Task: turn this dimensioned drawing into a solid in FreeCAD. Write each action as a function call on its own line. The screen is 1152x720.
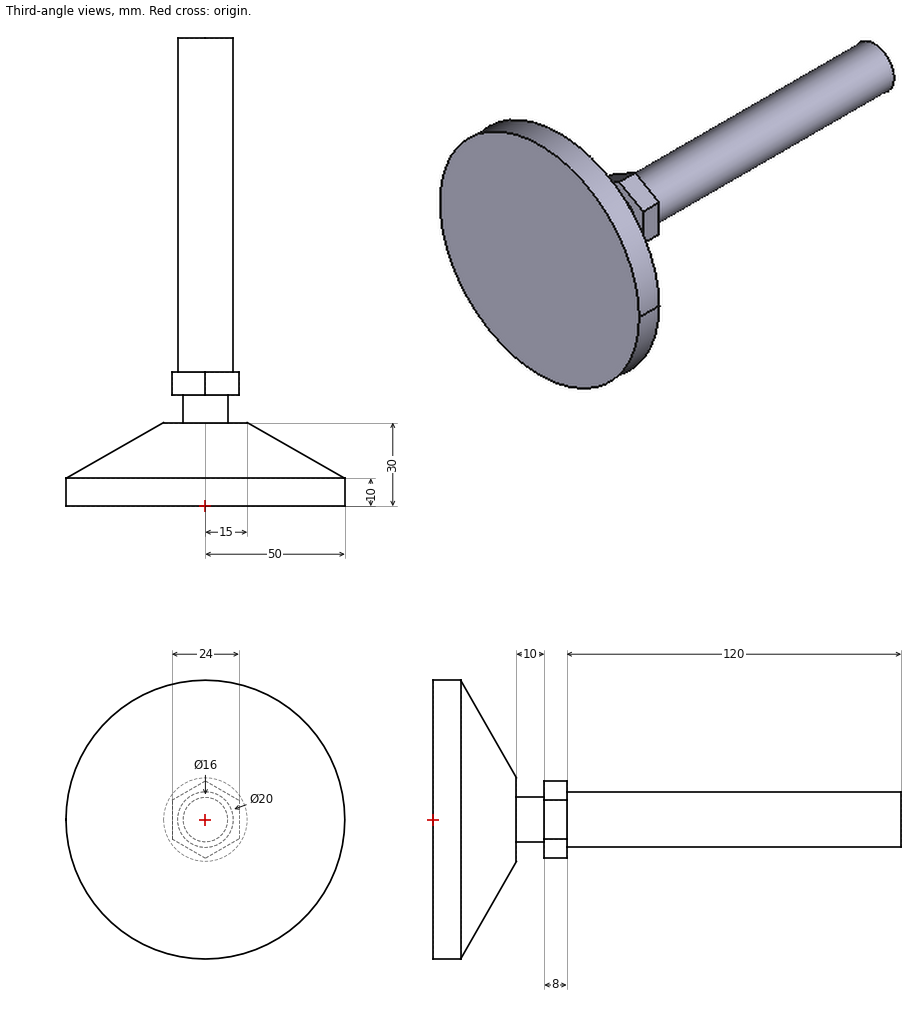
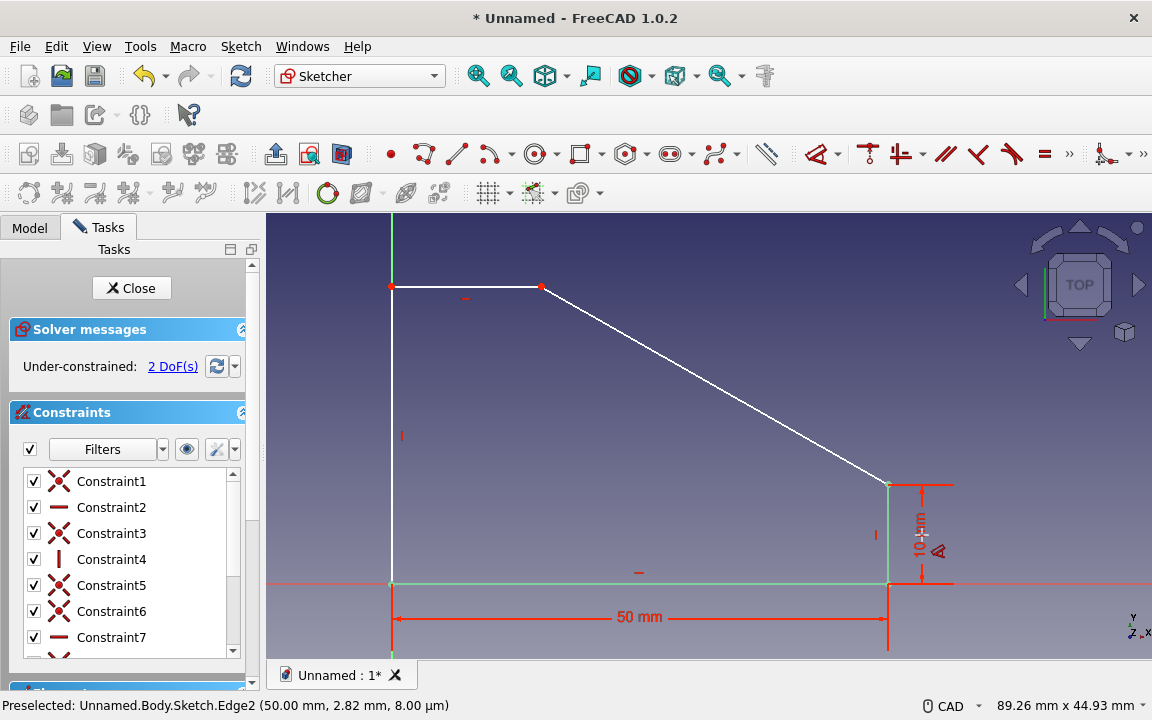
click(496, 287)
click(466, 253)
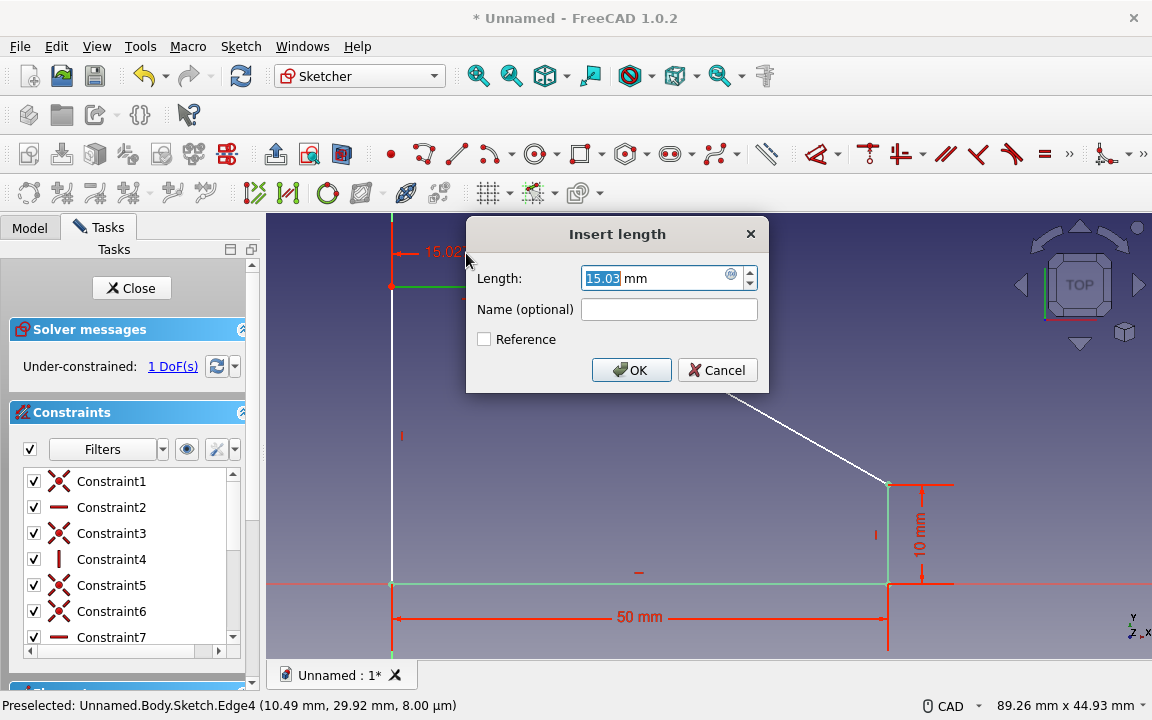
text(15)
key(Return)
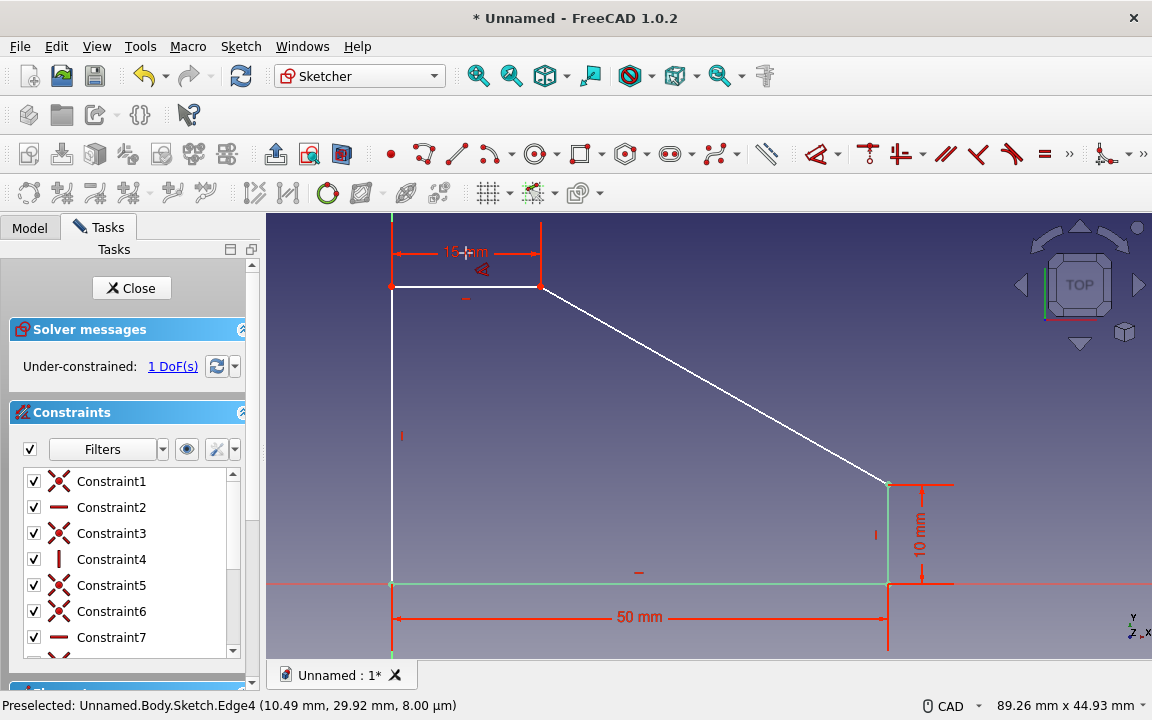
click(392, 376)
click(358, 436)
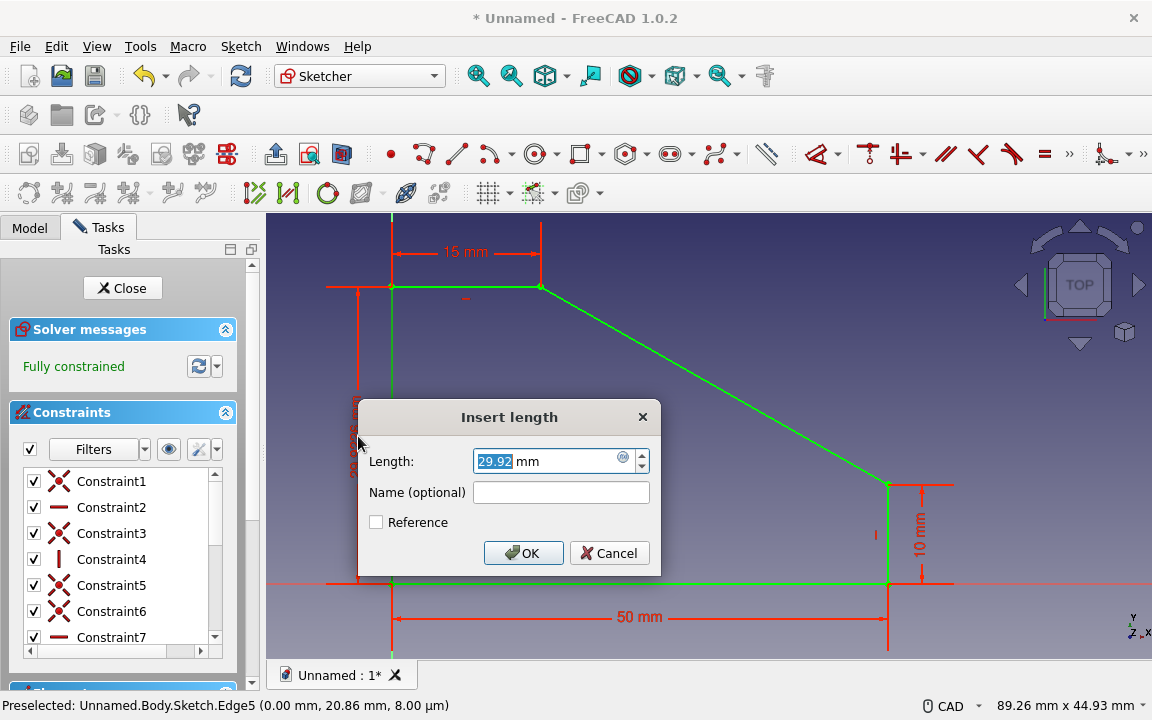
text(30)
key(Return)
key(Escape)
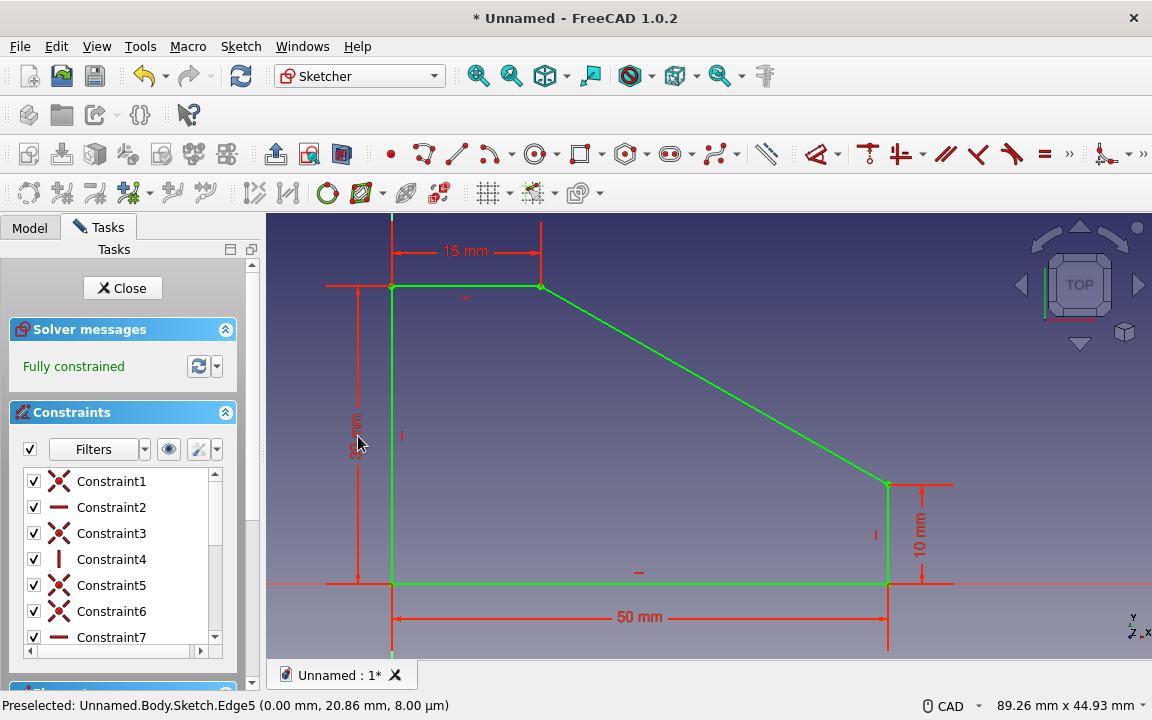
click(123, 288)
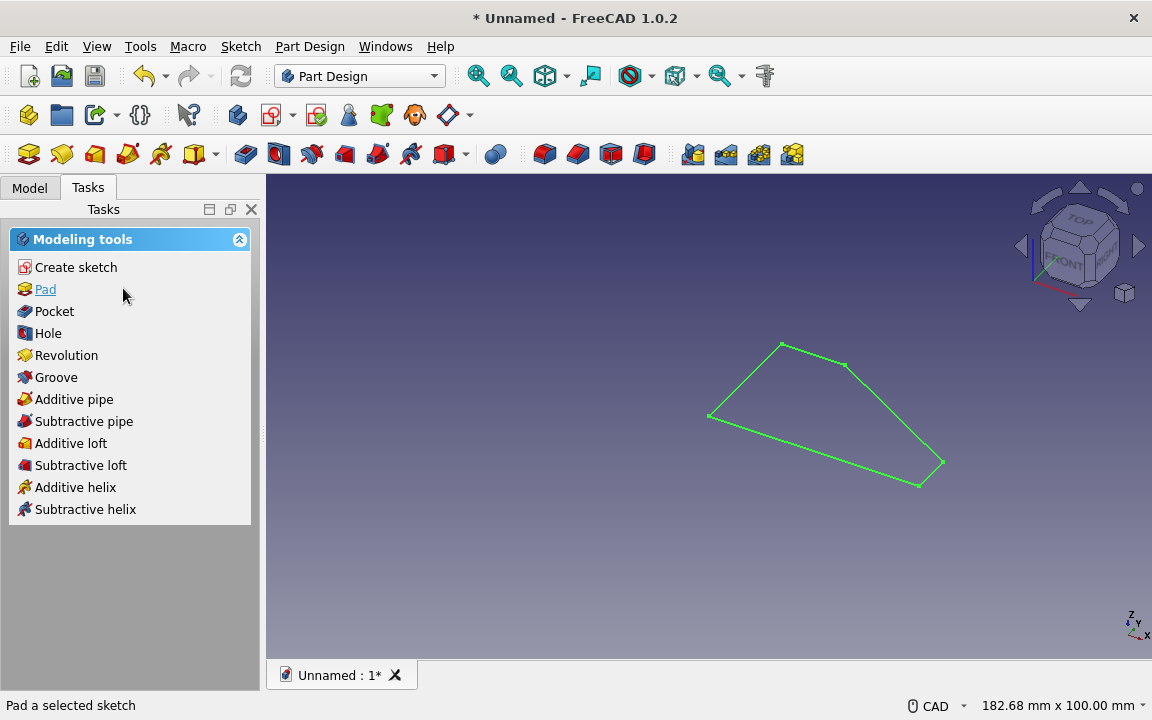
click(62, 154)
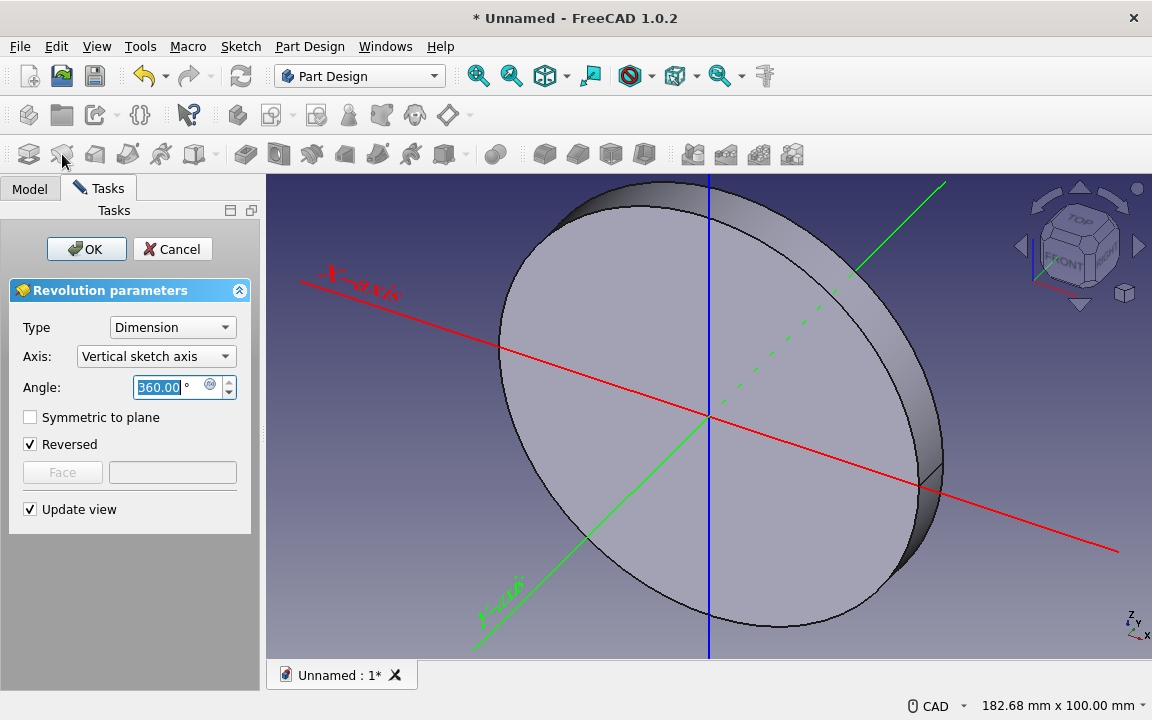
click(87, 249)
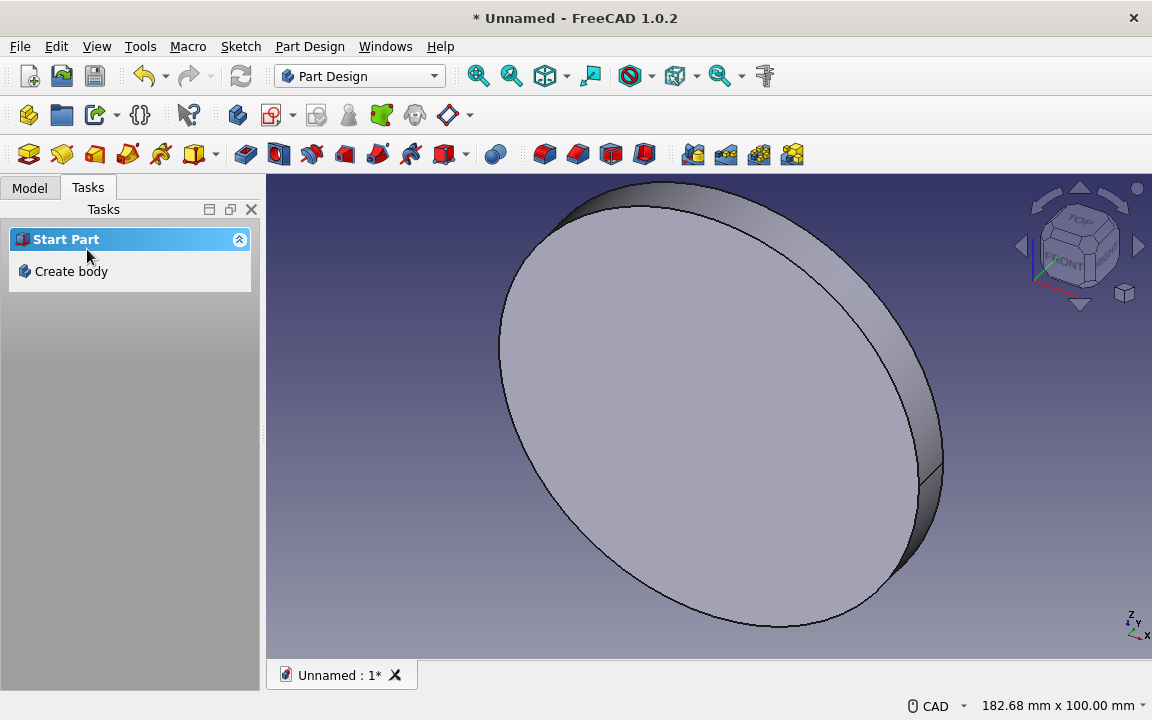
click(479, 76)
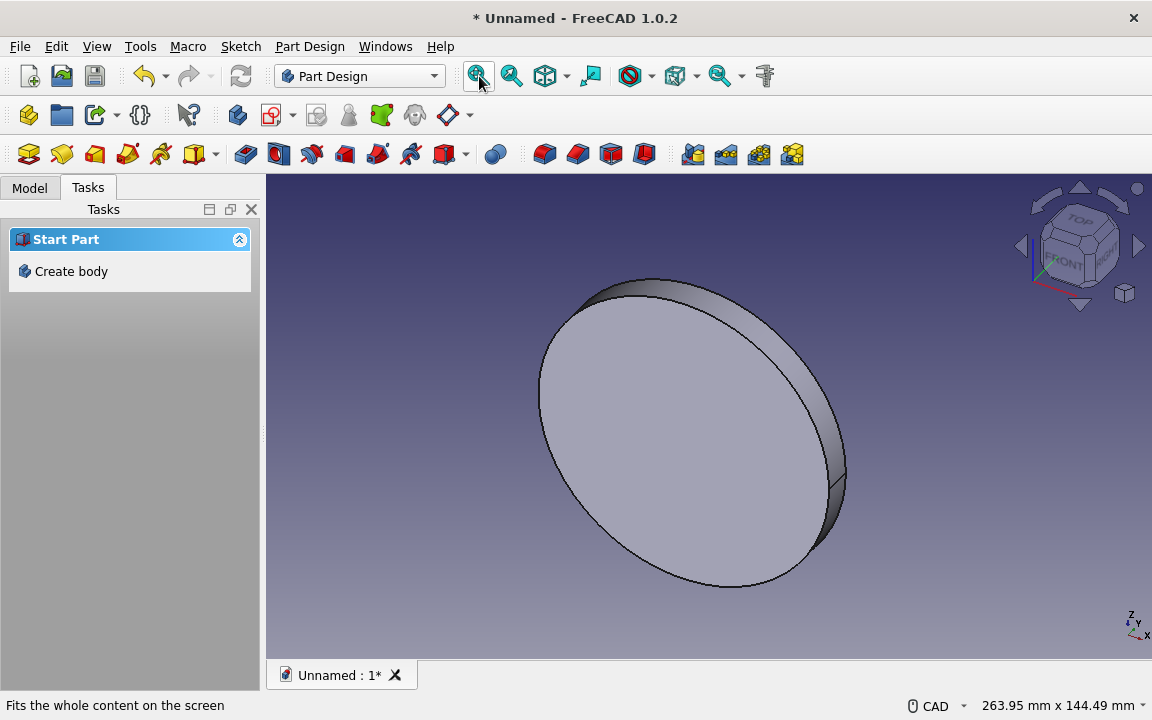
key(4)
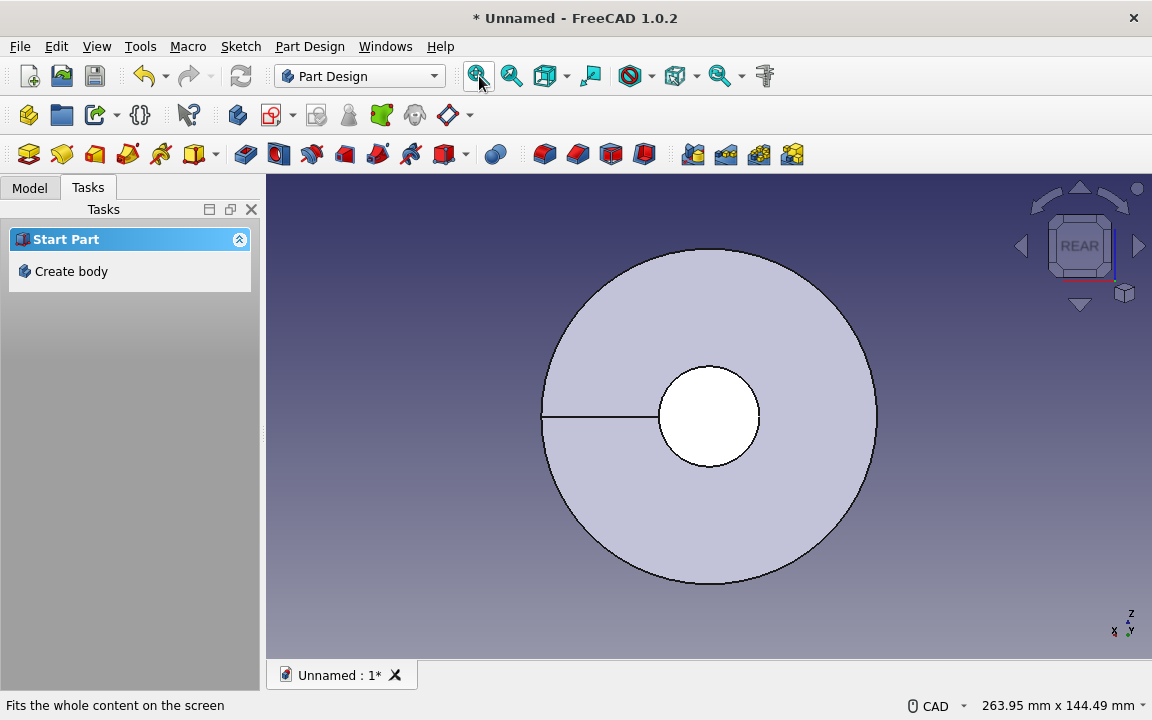
click(709, 415)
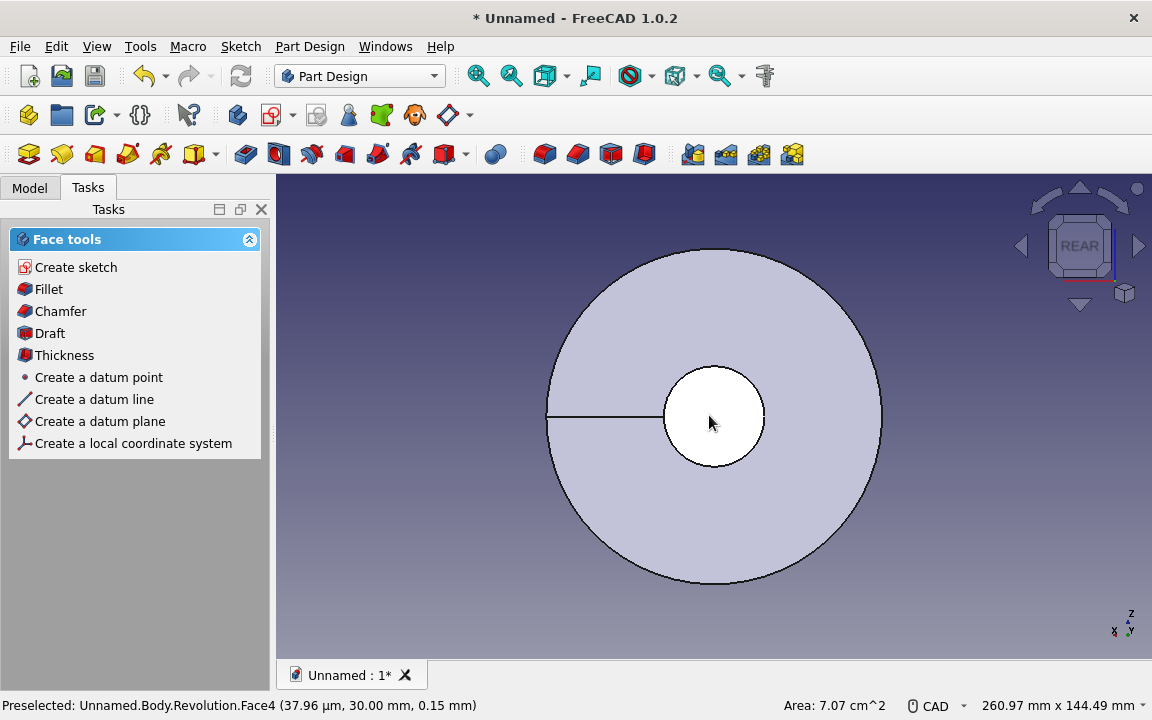
click(270, 116)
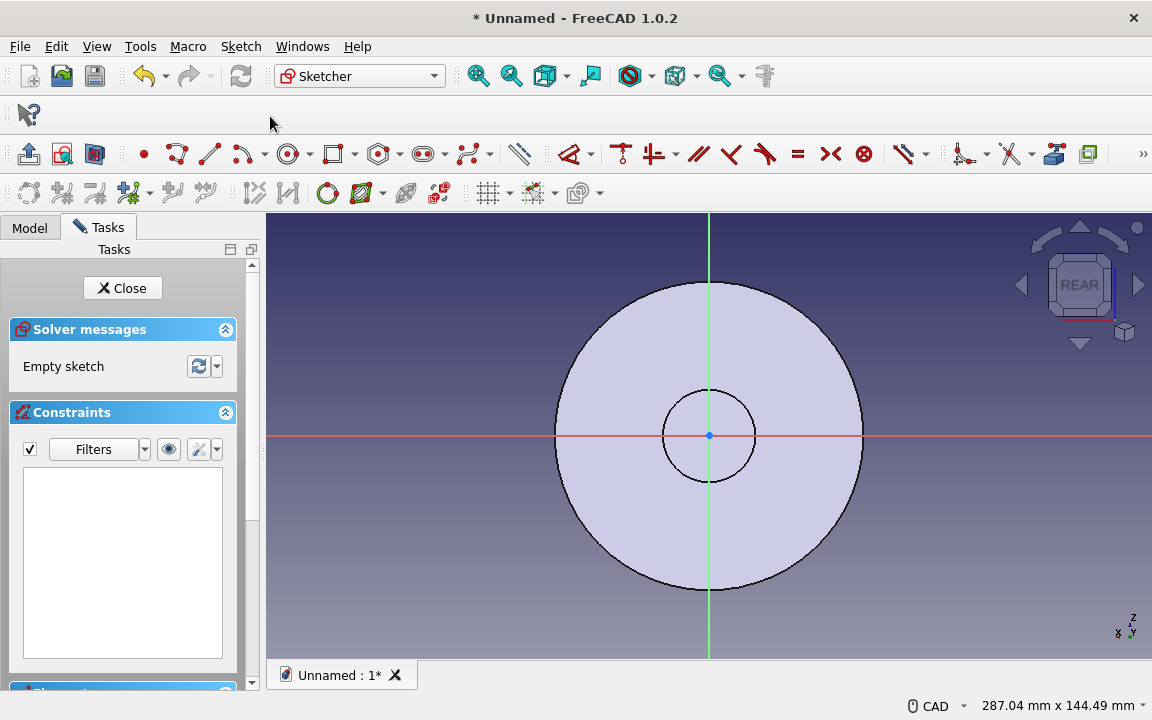
scroll(723, 436, up, 9)